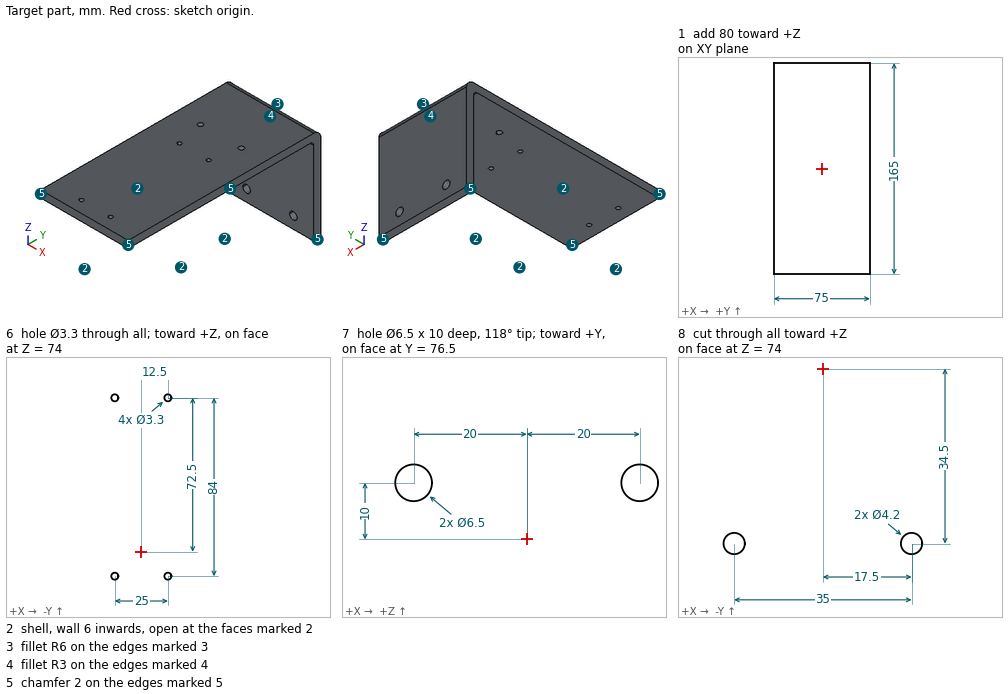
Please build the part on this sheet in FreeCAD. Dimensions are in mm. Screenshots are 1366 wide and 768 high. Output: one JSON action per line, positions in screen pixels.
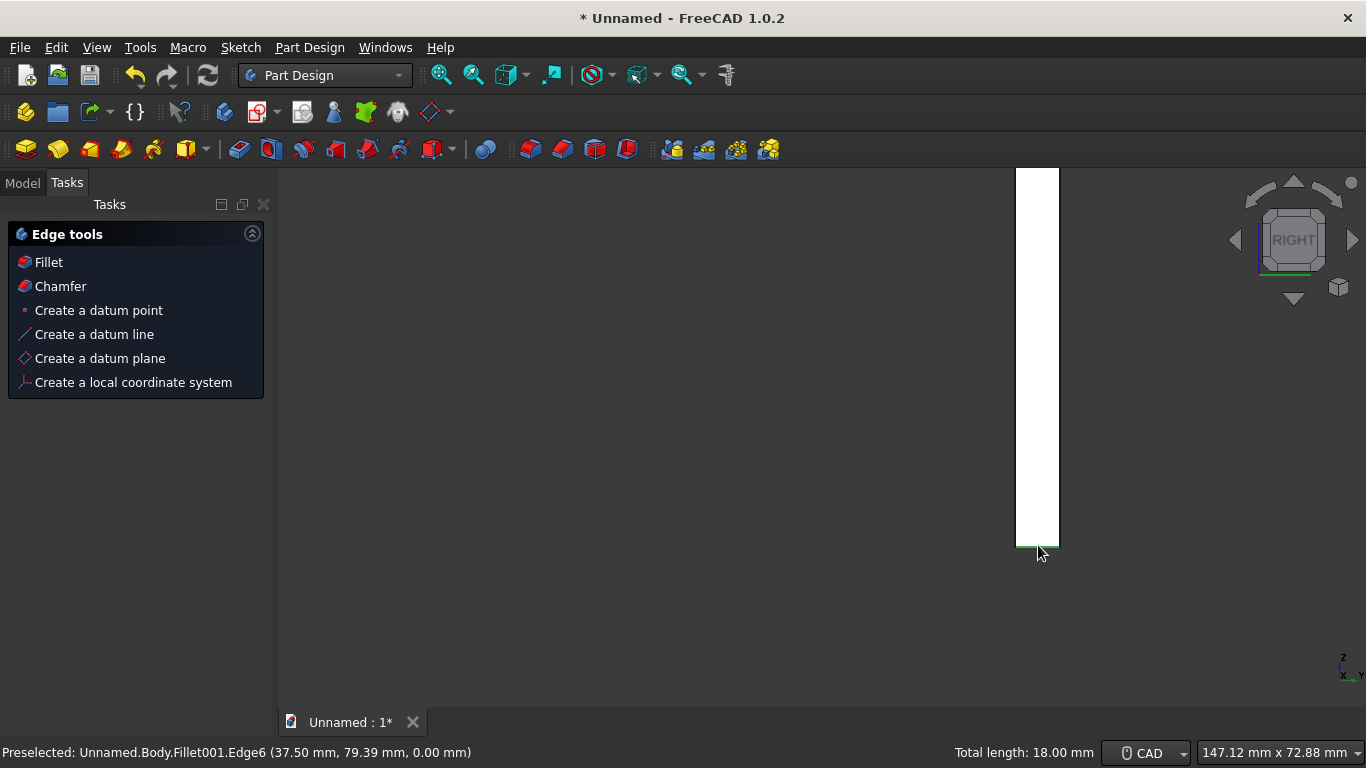
{"action": "left_click", "coordinate": [442, 76]}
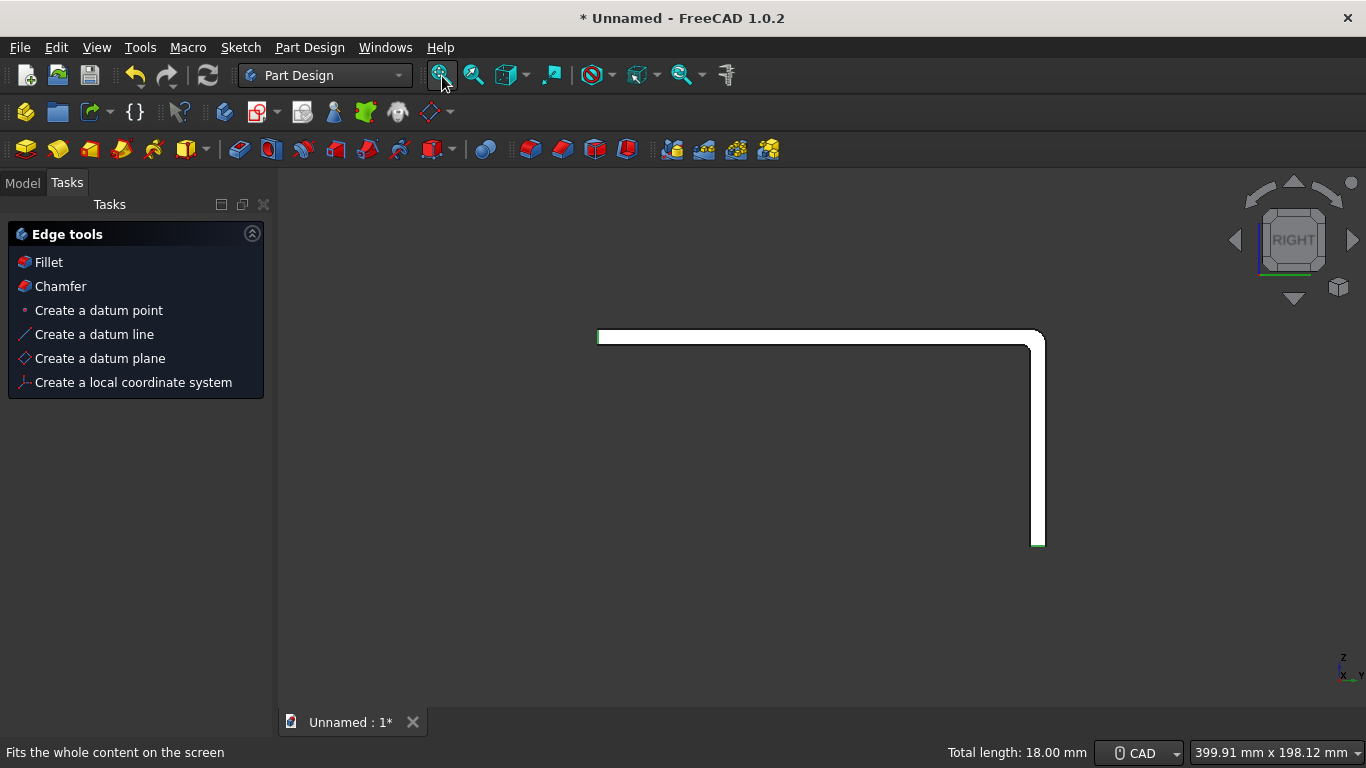
{"action": "key", "text": "5"}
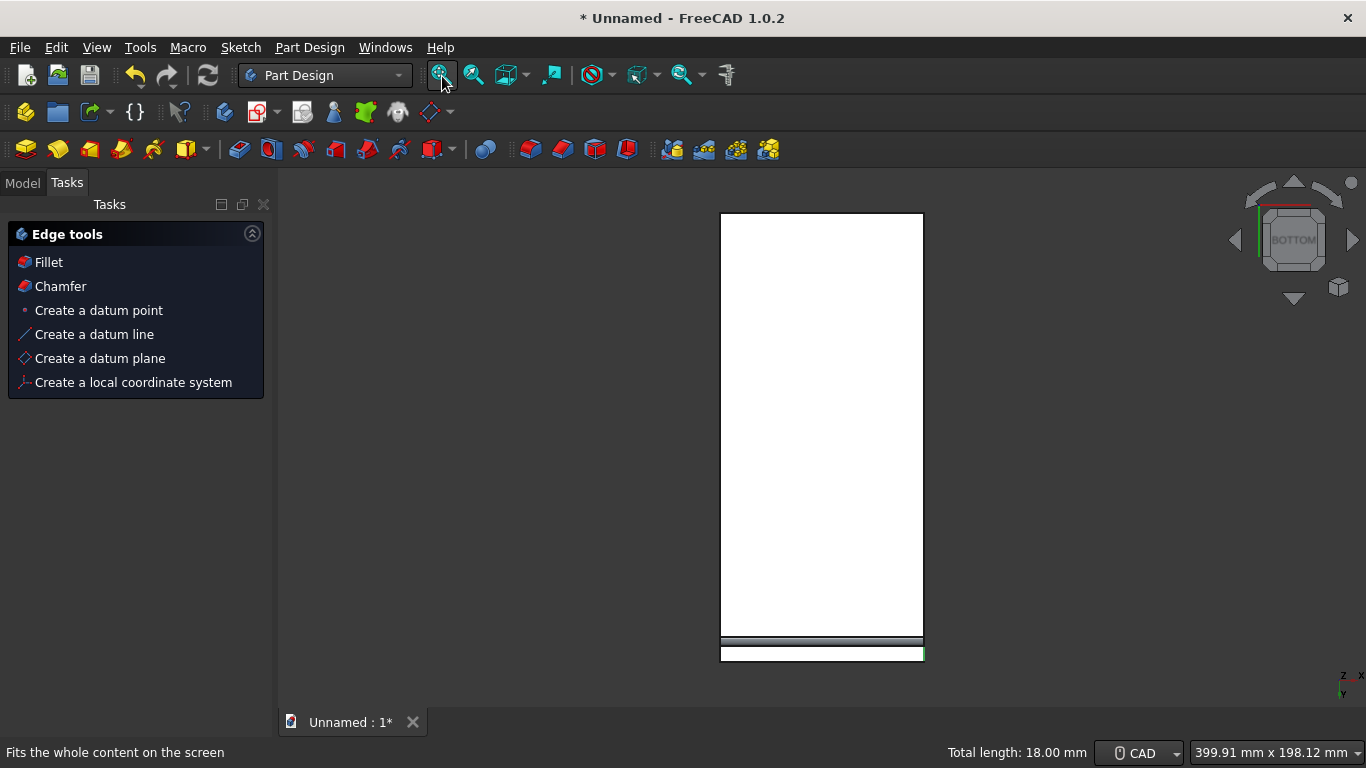
{"action": "left_click", "coordinate": [720, 653], "text": "ctrl"}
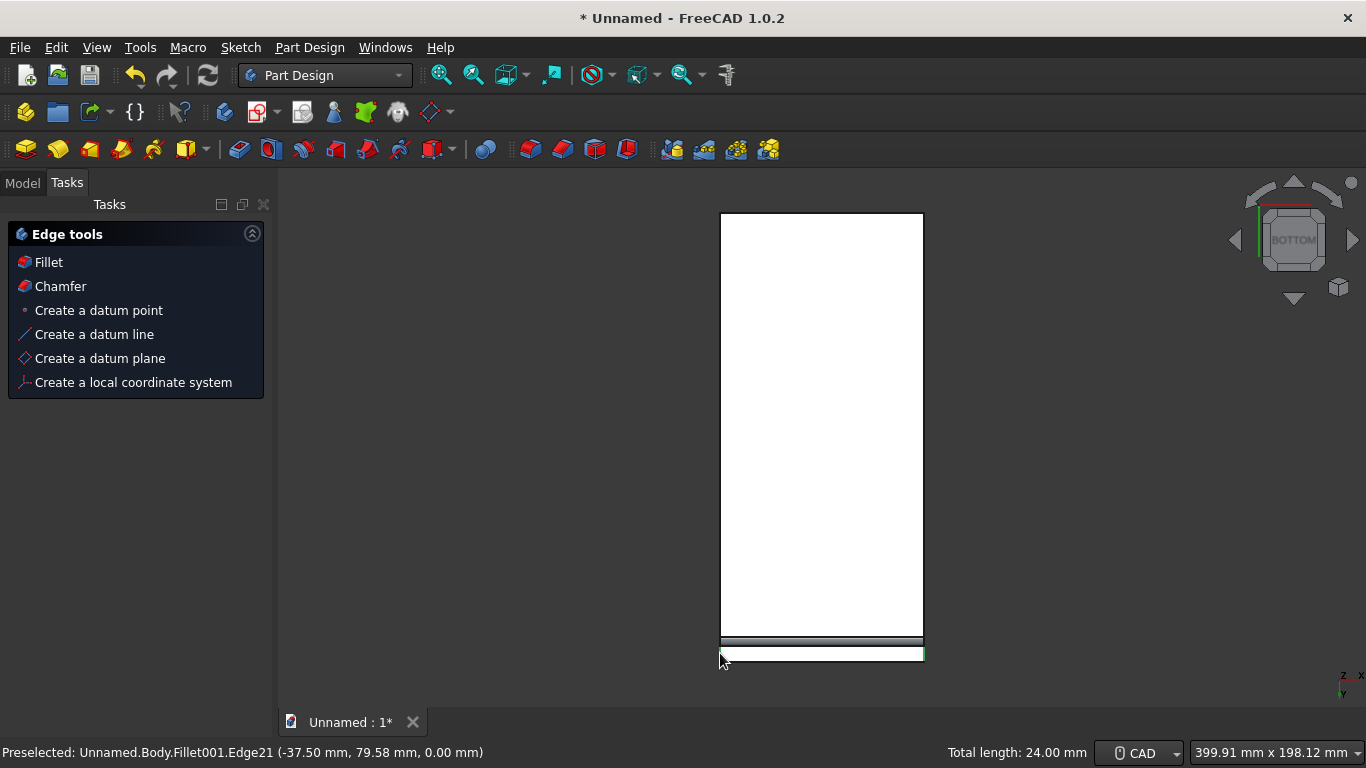
{"action": "left_click", "coordinate": [564, 150]}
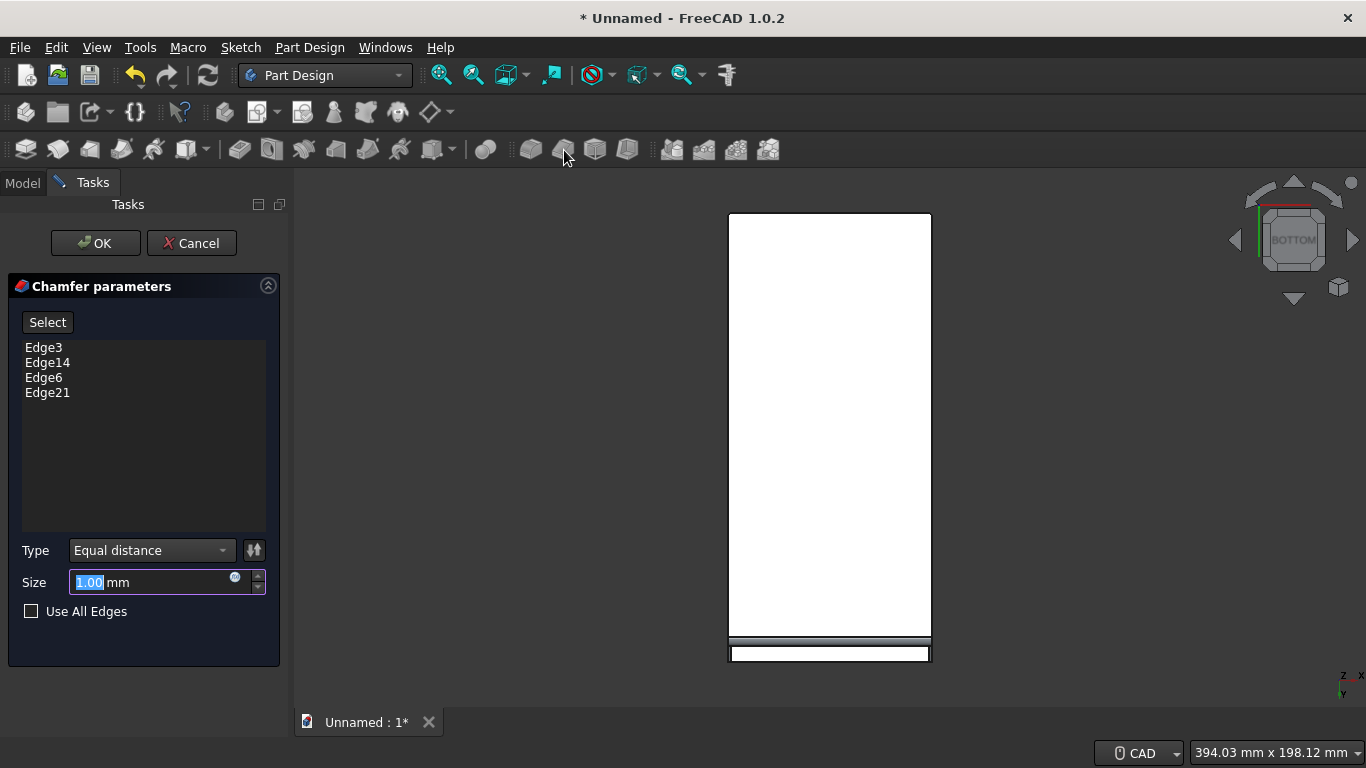
{"action": "type", "text": "2"}
{"action": "key", "text": "Tab"}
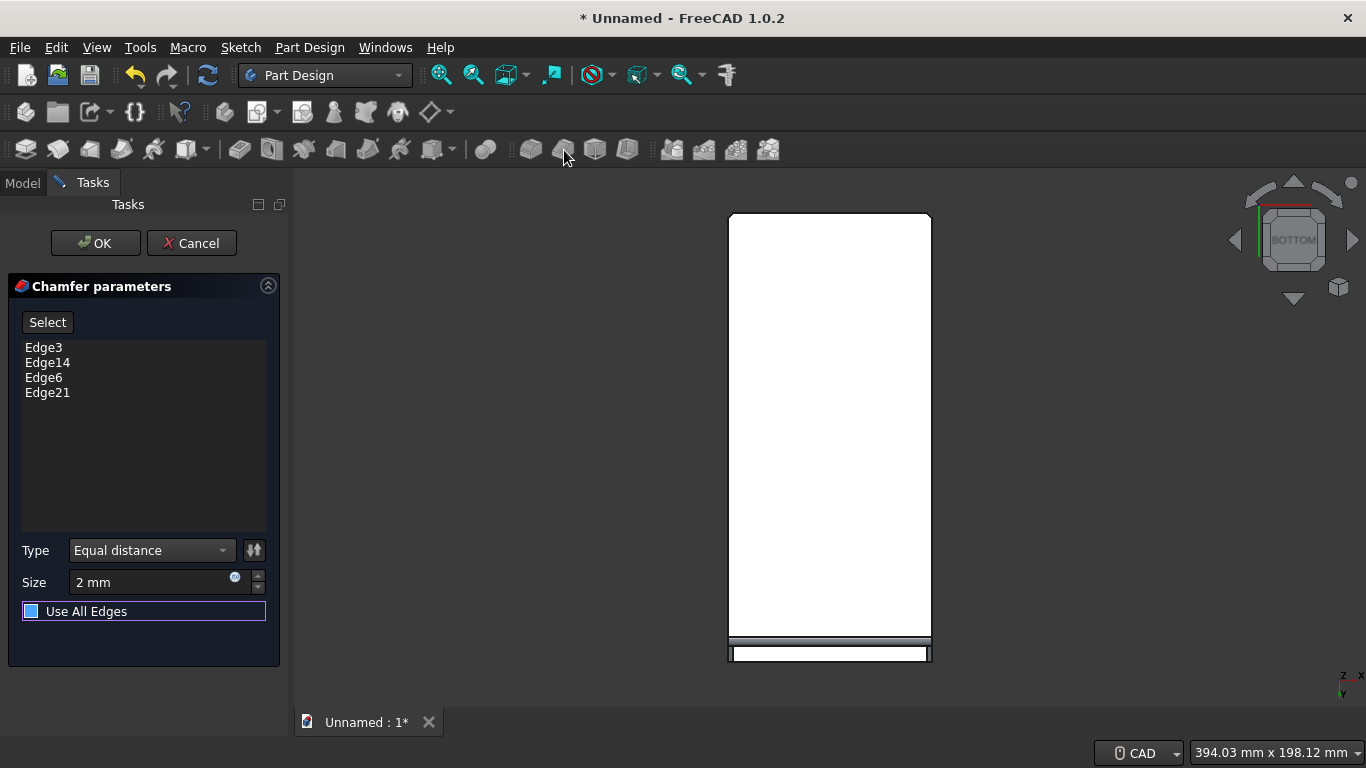
{"action": "left_click", "coordinate": [96, 243]}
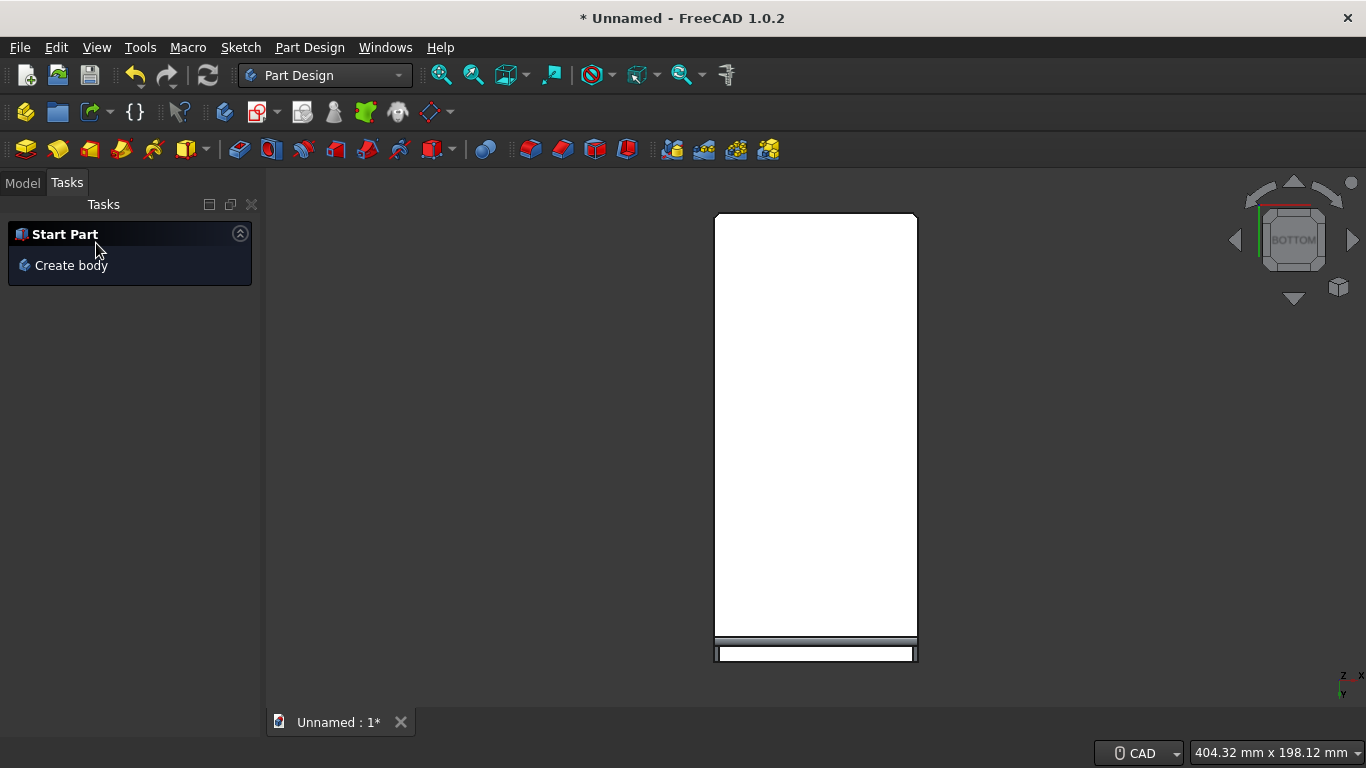
{"action": "left_click", "coordinate": [816, 485]}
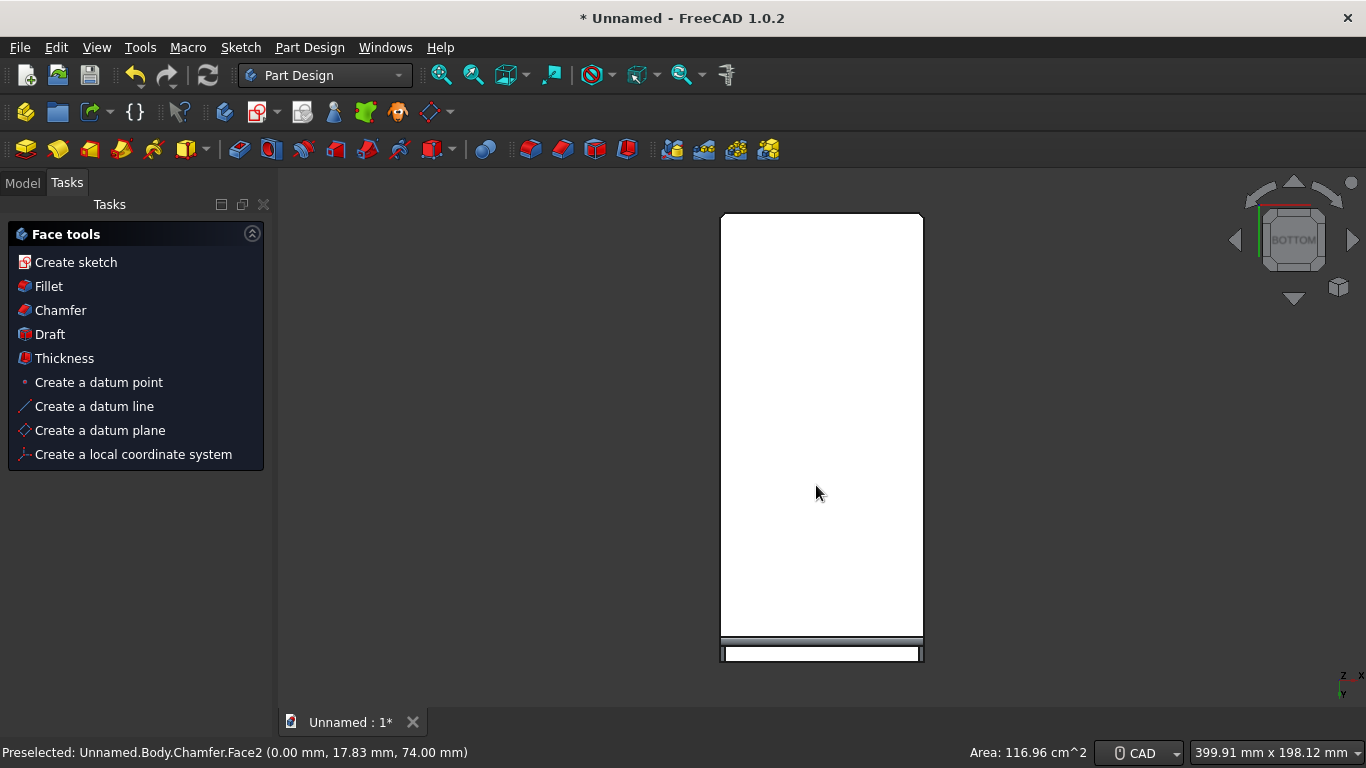
{"action": "left_click", "coordinate": [258, 112]}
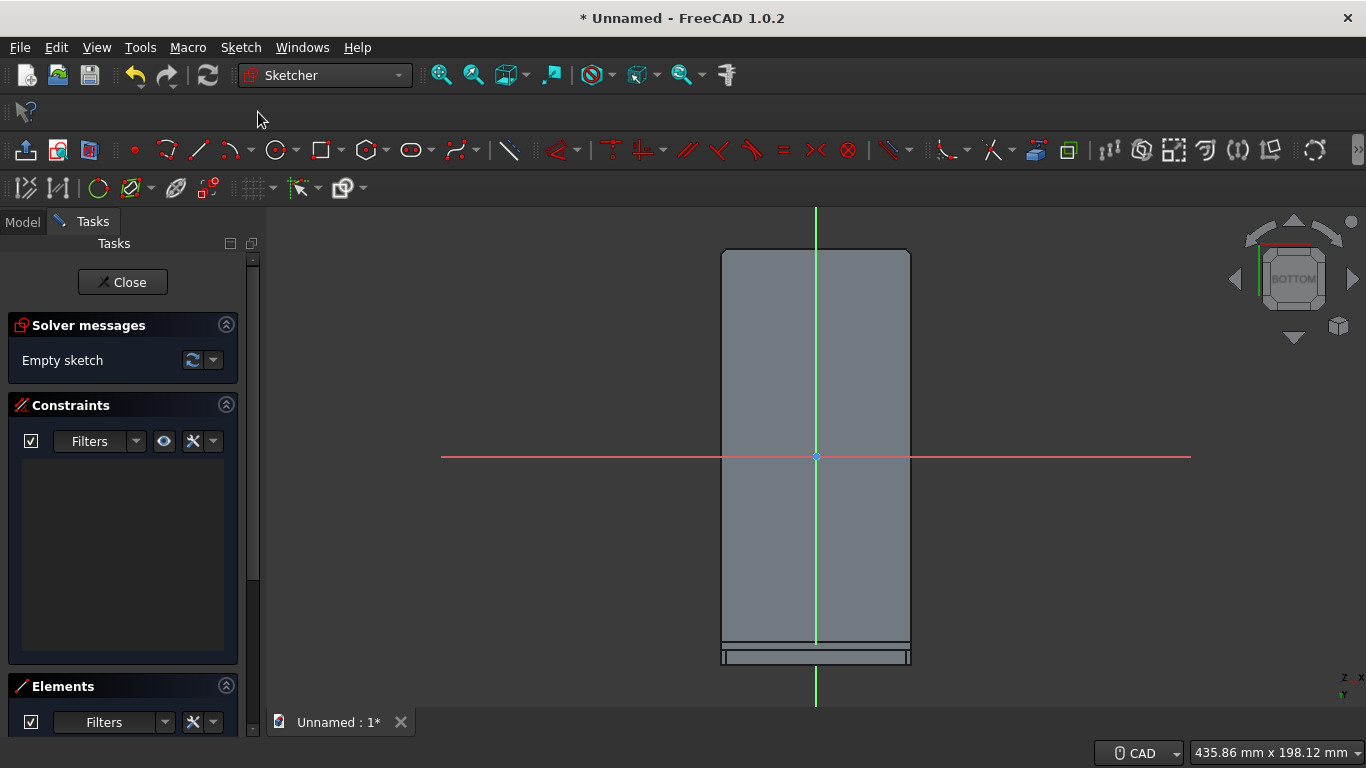
{"action": "scroll", "coordinate": [955, 235], "scroll_direction": "up", "scroll_amount": 2}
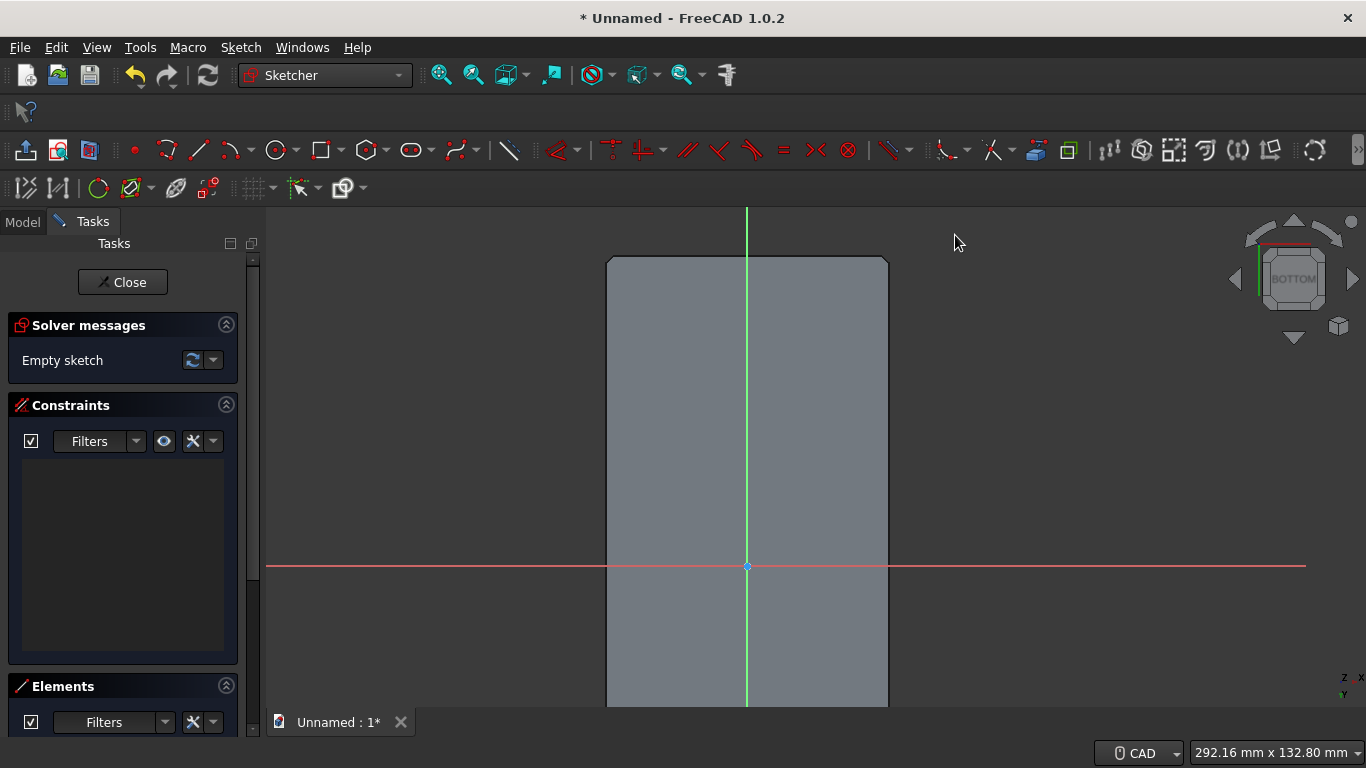
{"action": "left_click", "coordinate": [276, 150]}